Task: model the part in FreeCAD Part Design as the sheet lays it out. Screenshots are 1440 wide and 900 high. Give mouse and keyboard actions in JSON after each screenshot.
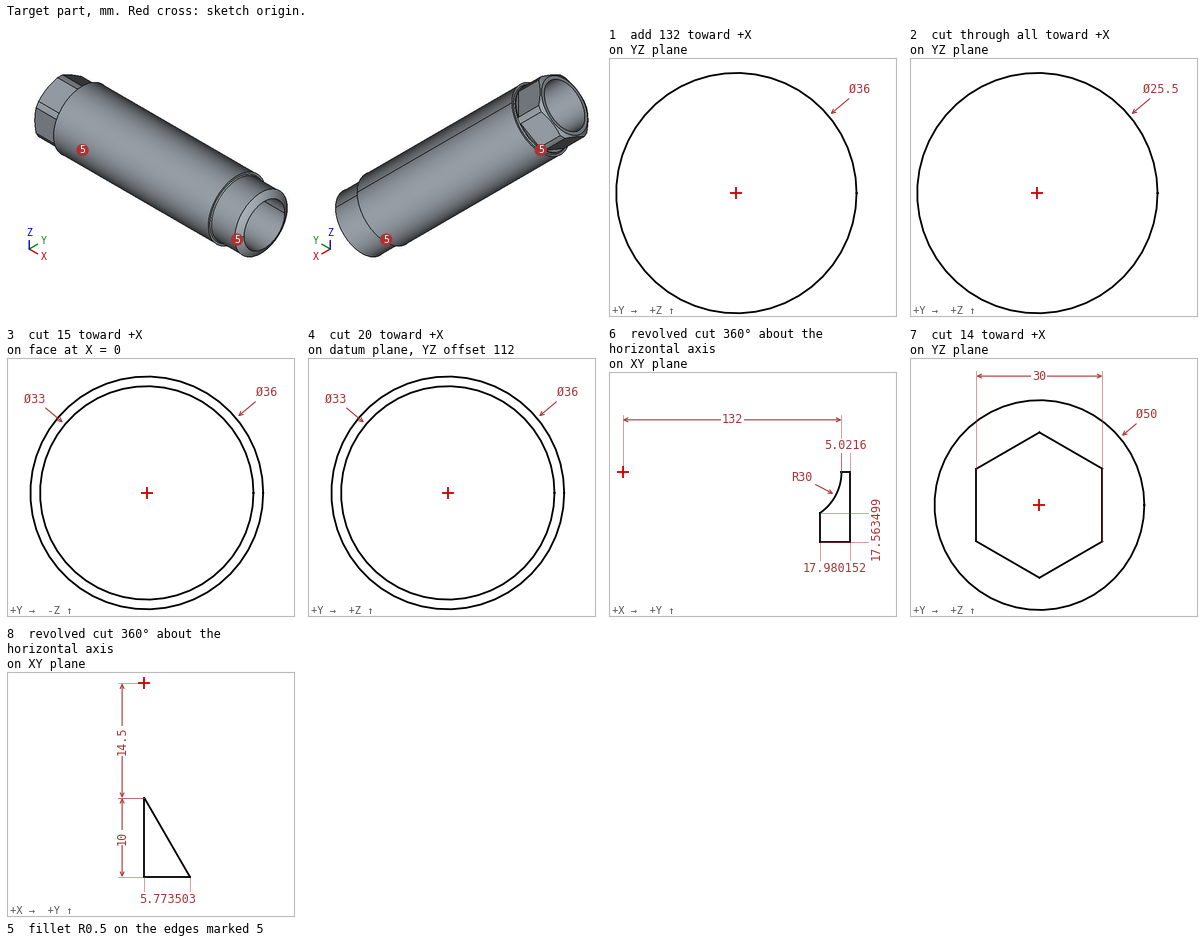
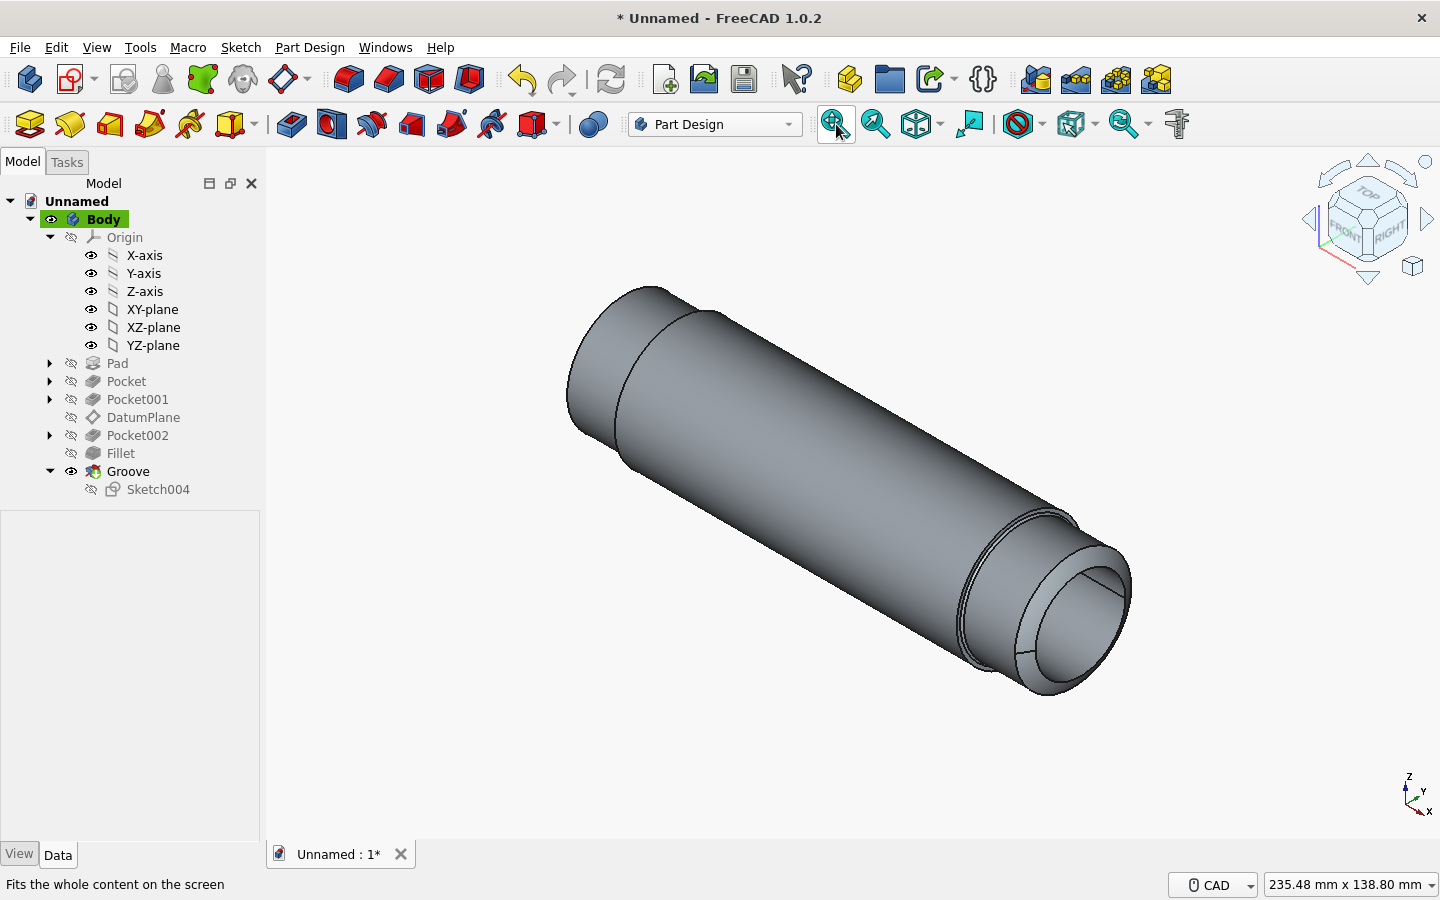
{"action": "left_click", "coordinate": [70, 80]}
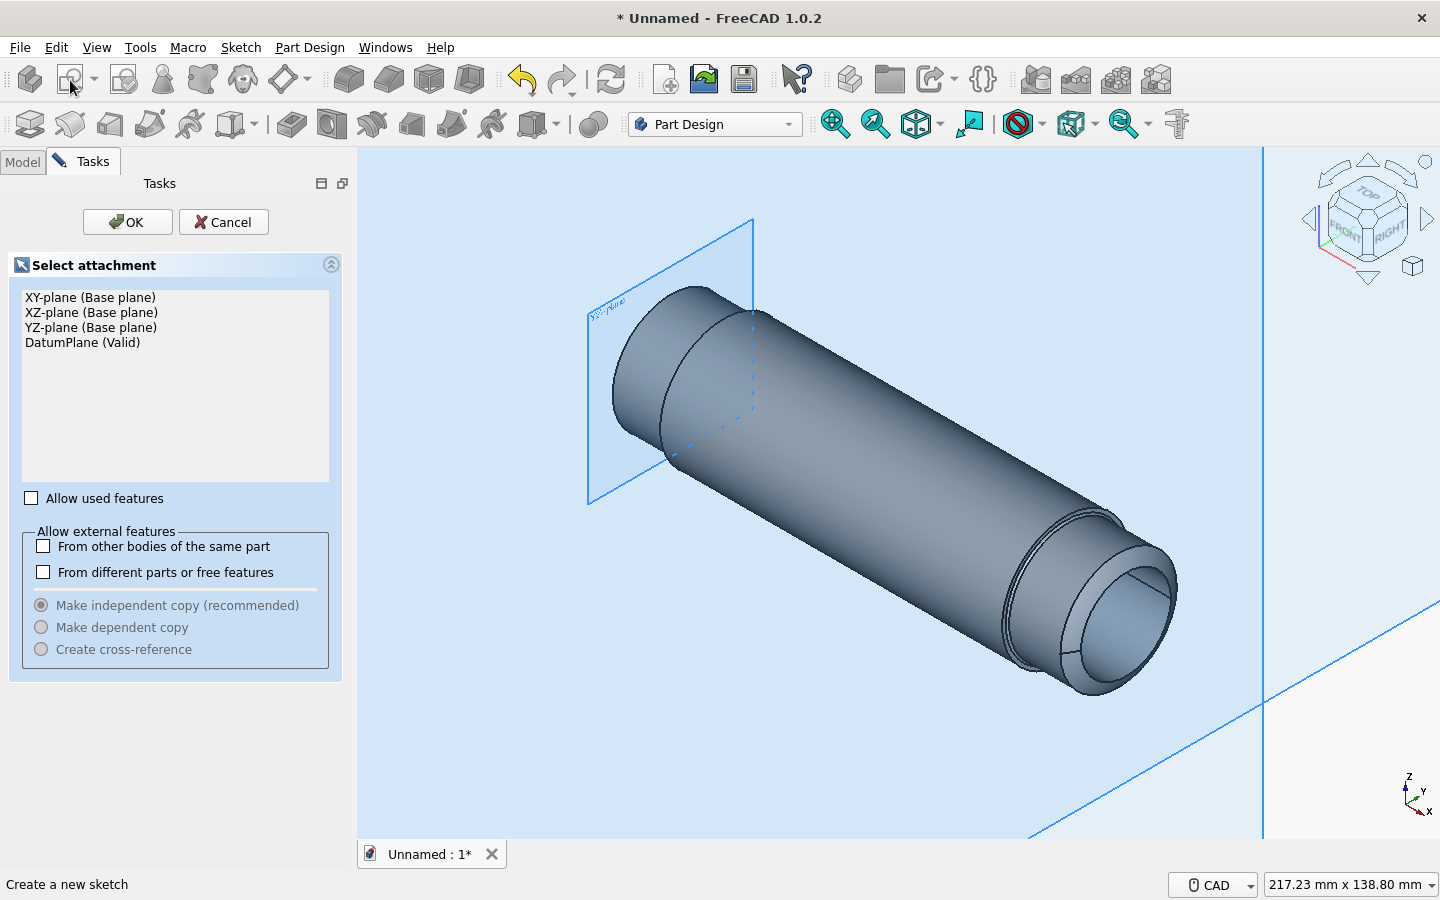
{"action": "left_click", "coordinate": [82, 328]}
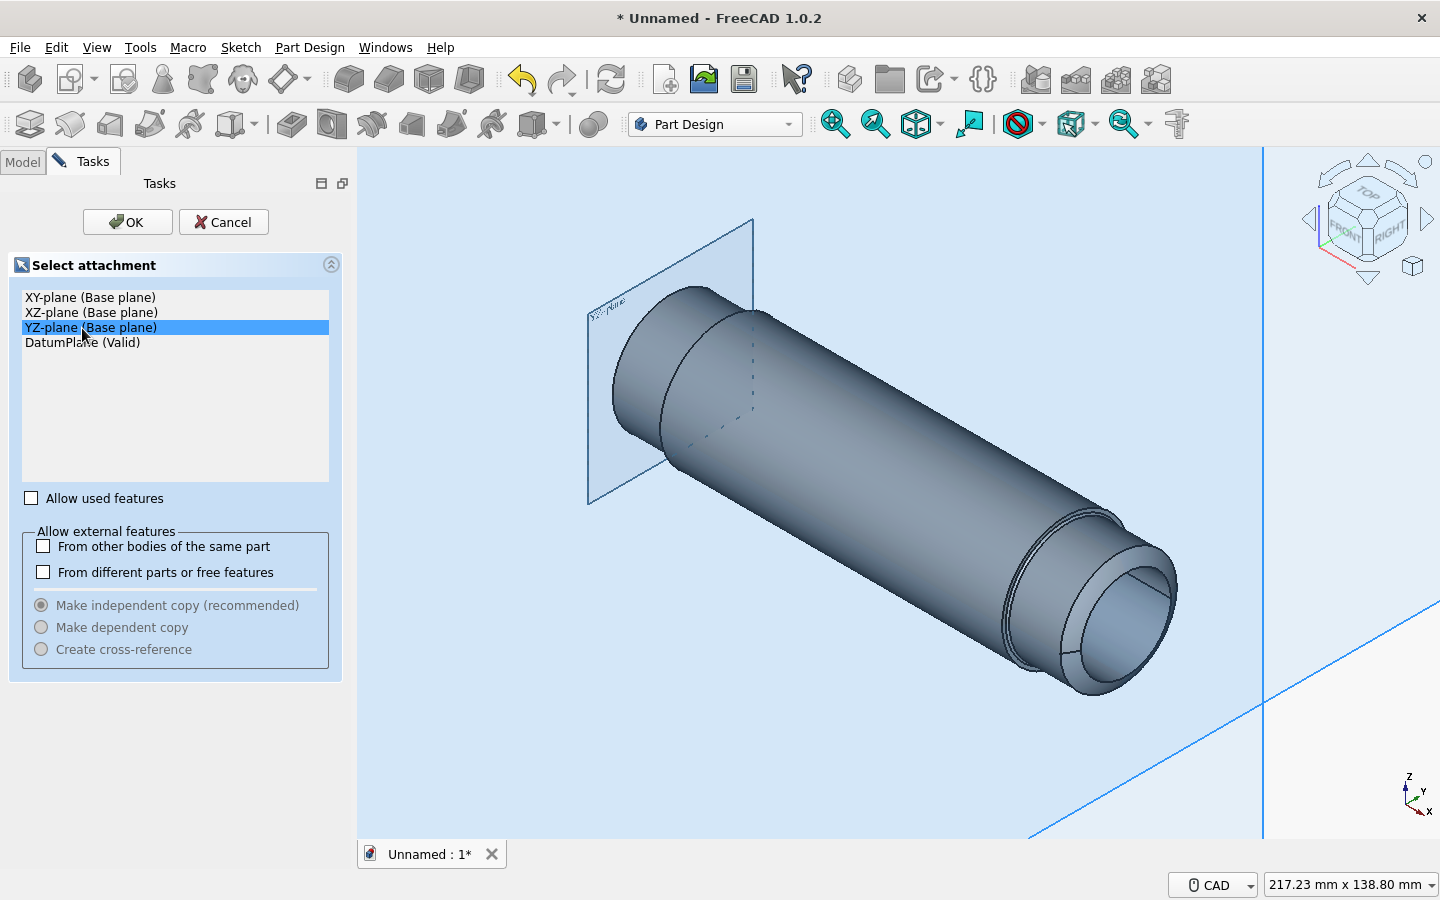
{"action": "left_click", "coordinate": [128, 222]}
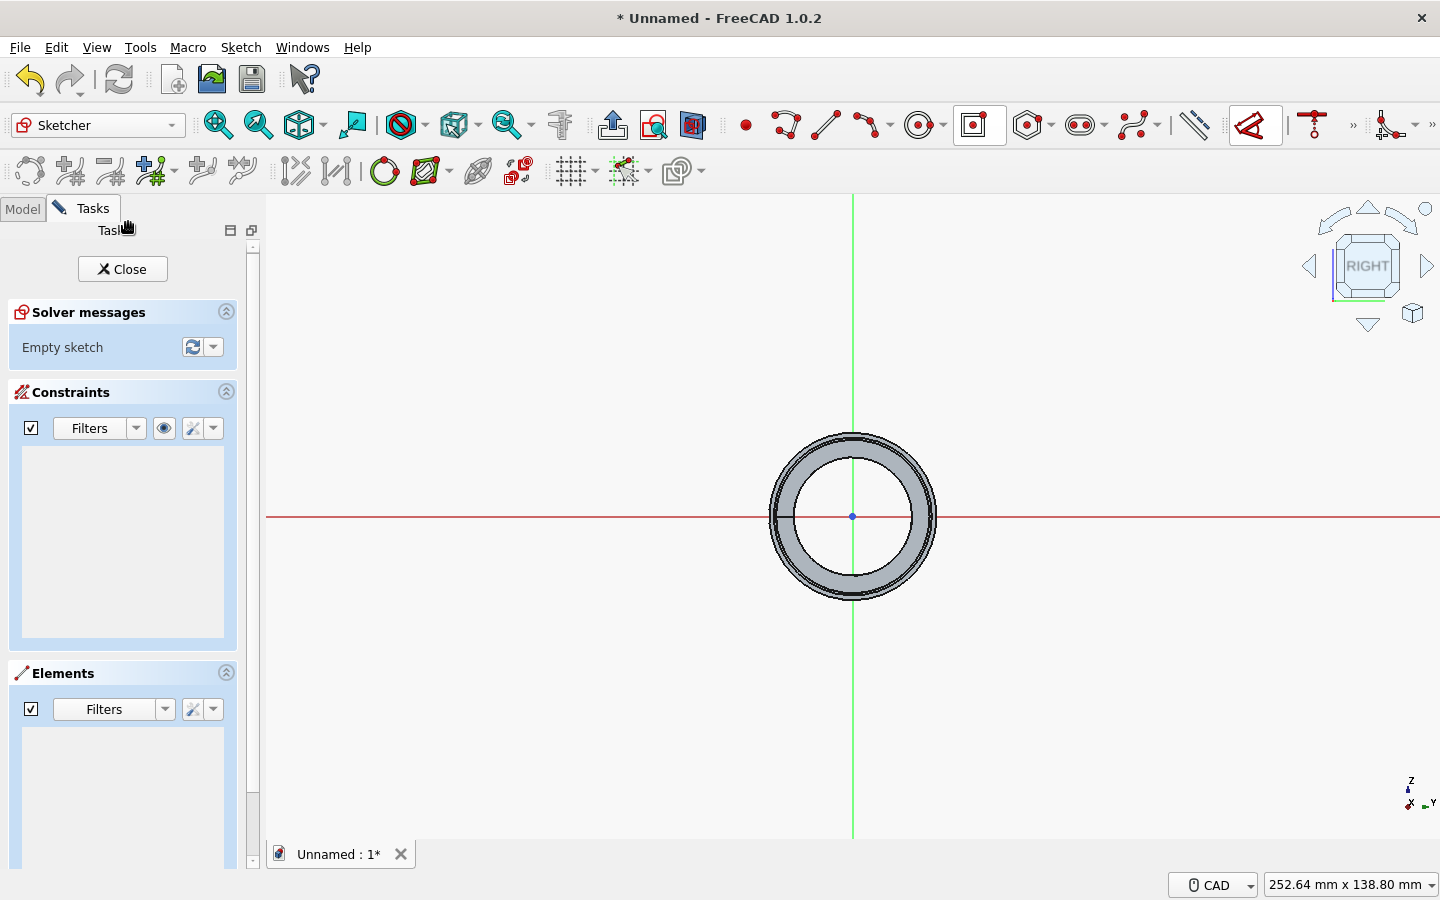
{"action": "left_click", "coordinate": [694, 126]}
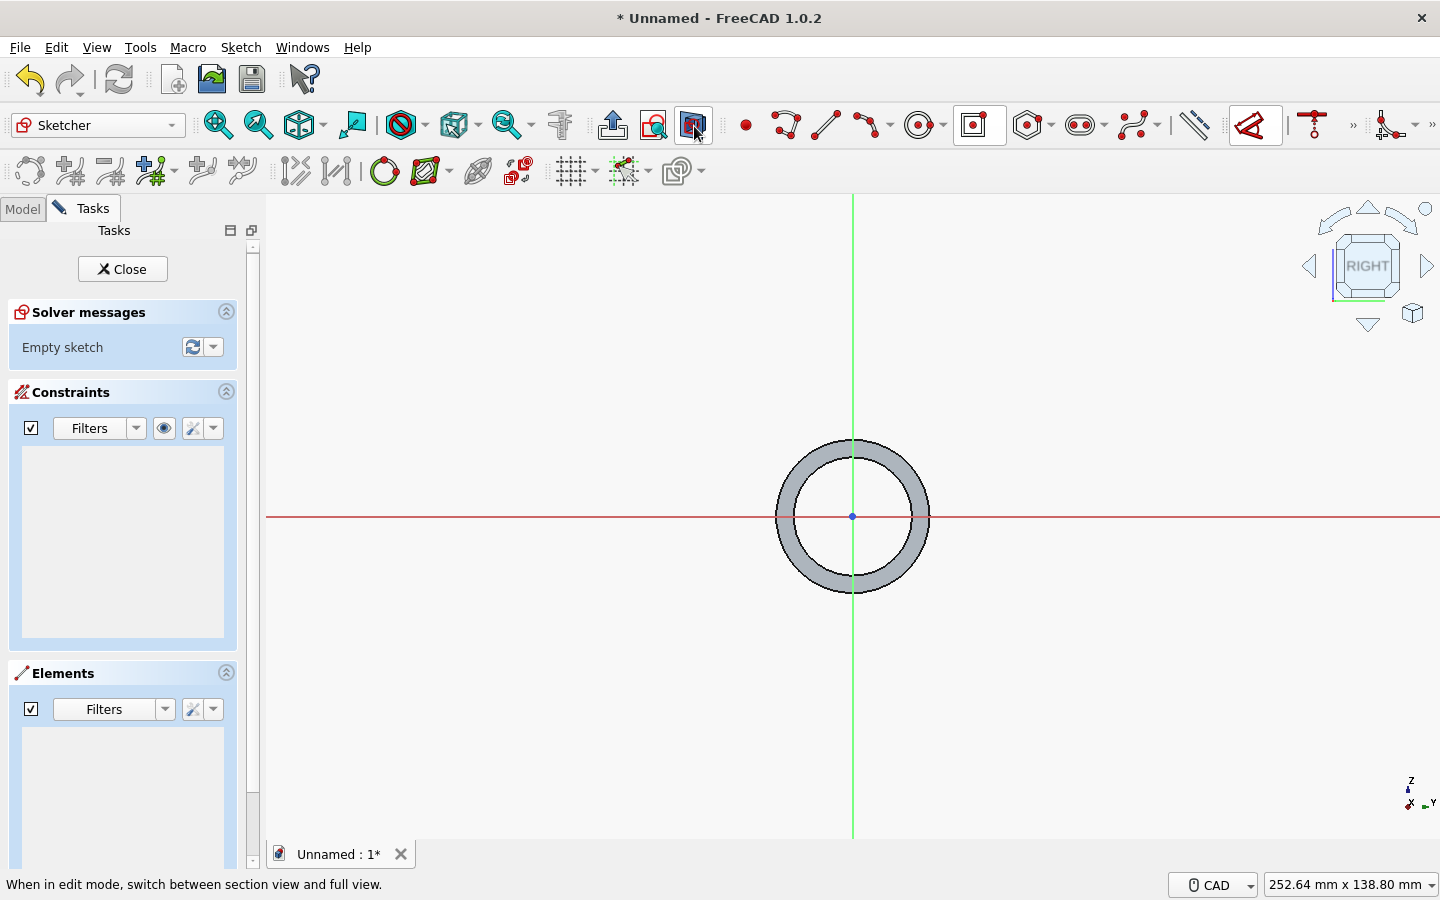
{"action": "scroll", "coordinate": [936, 516], "scroll_direction": "up", "scroll_amount": 3}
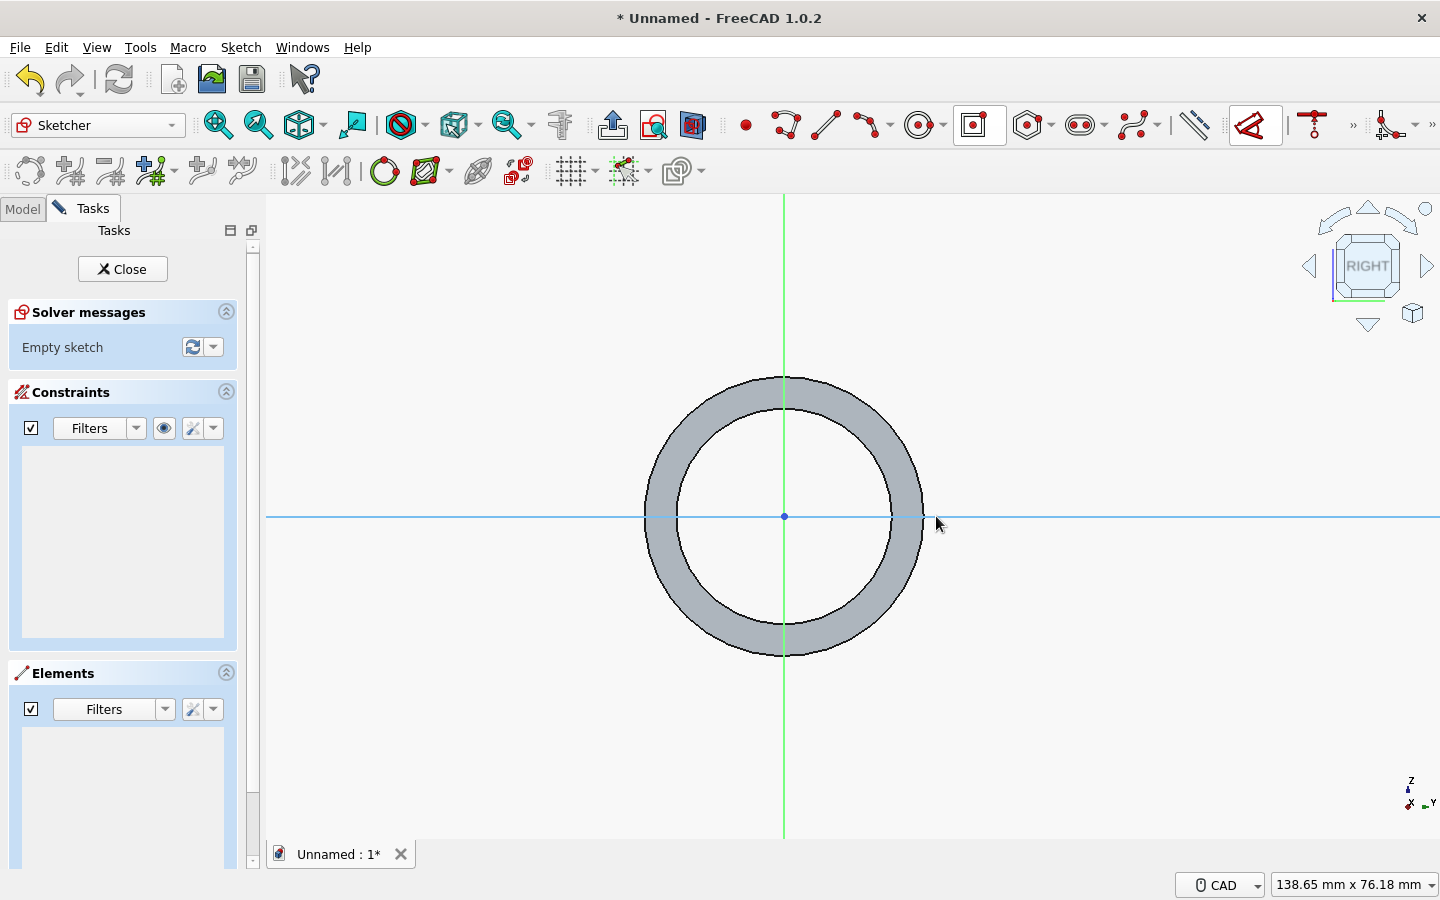
{"action": "left_click", "coordinate": [1028, 126]}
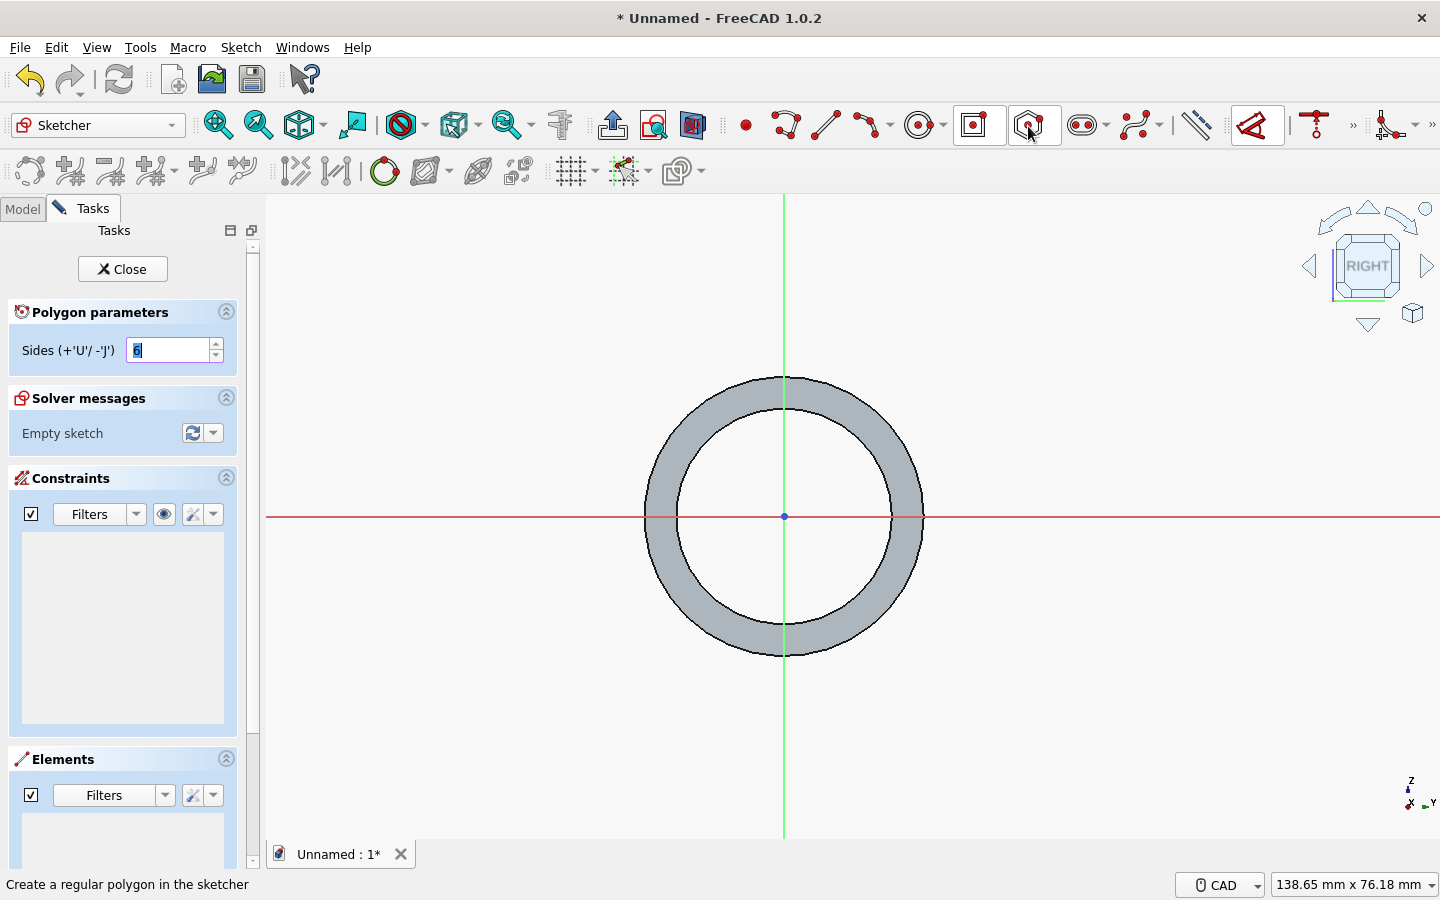
{"action": "left_click", "coordinate": [784, 516]}